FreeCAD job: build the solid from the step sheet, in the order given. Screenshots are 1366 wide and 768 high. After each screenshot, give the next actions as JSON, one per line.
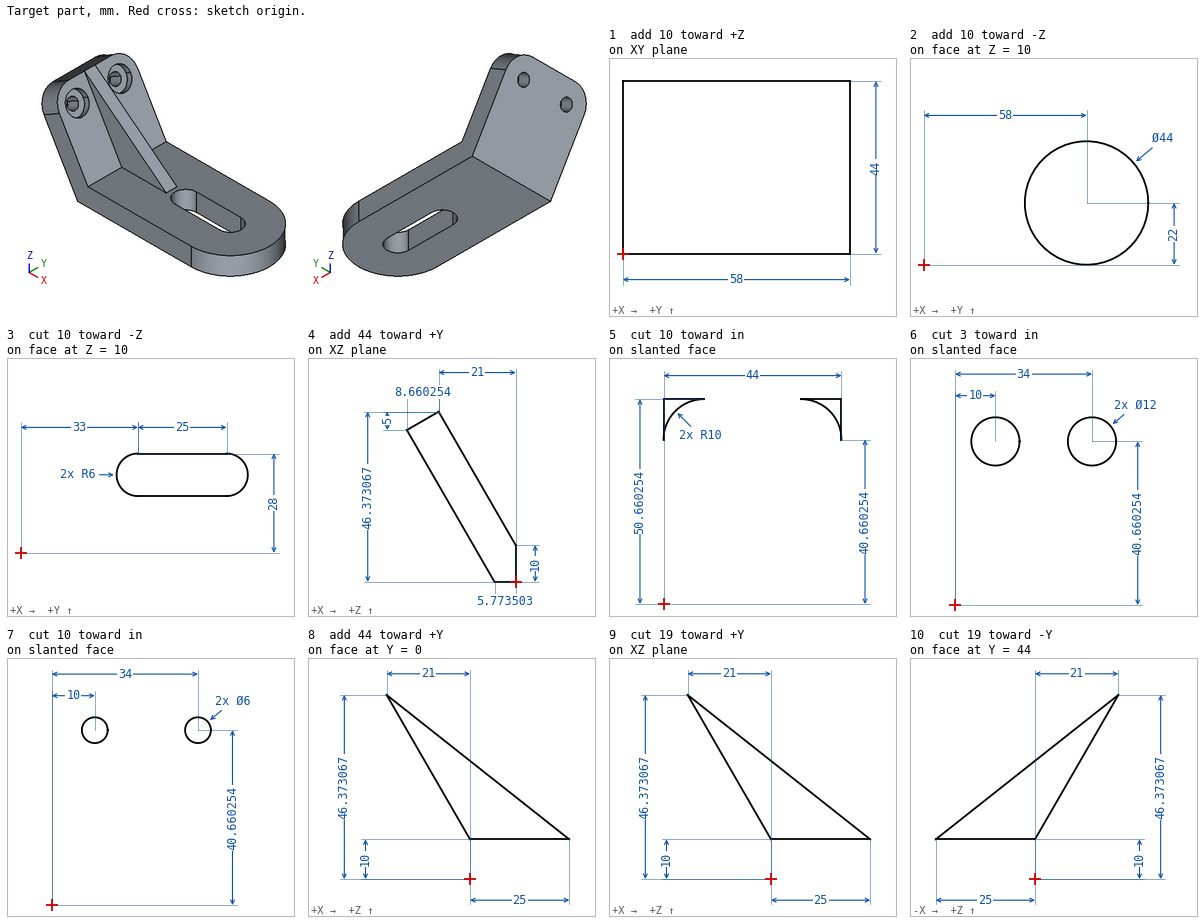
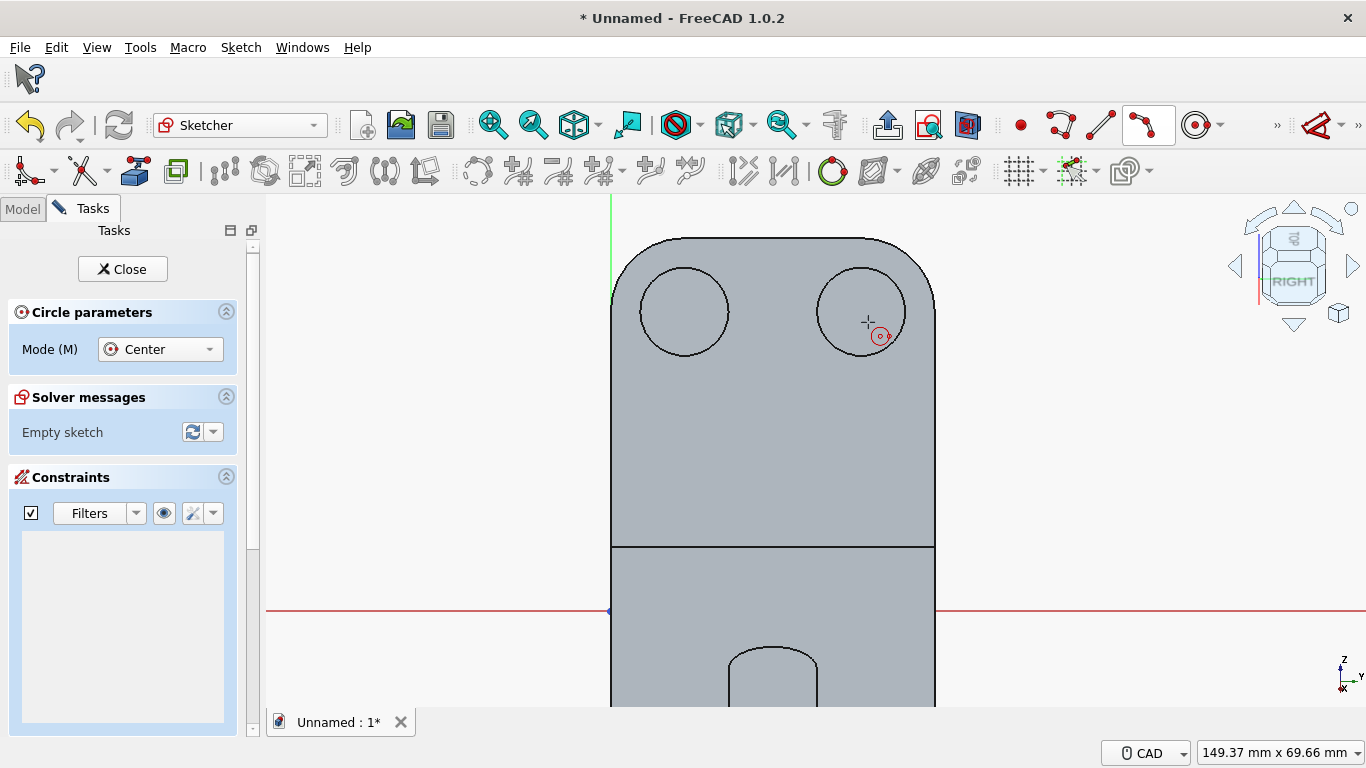
{"action": "left_click", "coordinate": [861, 312]}
{"action": "mouse_move", "coordinate": [877, 296]}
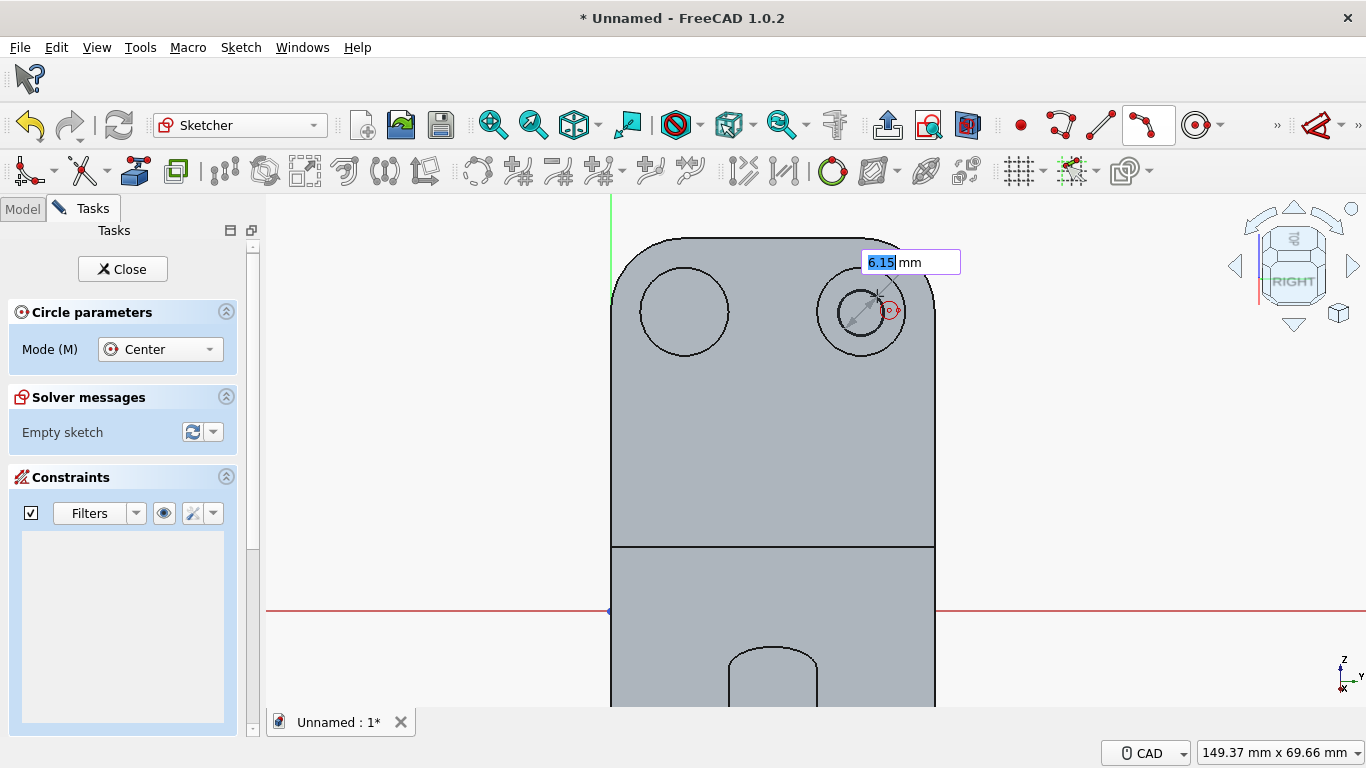
{"action": "type", "text": "6"}
{"action": "key", "text": "Return"}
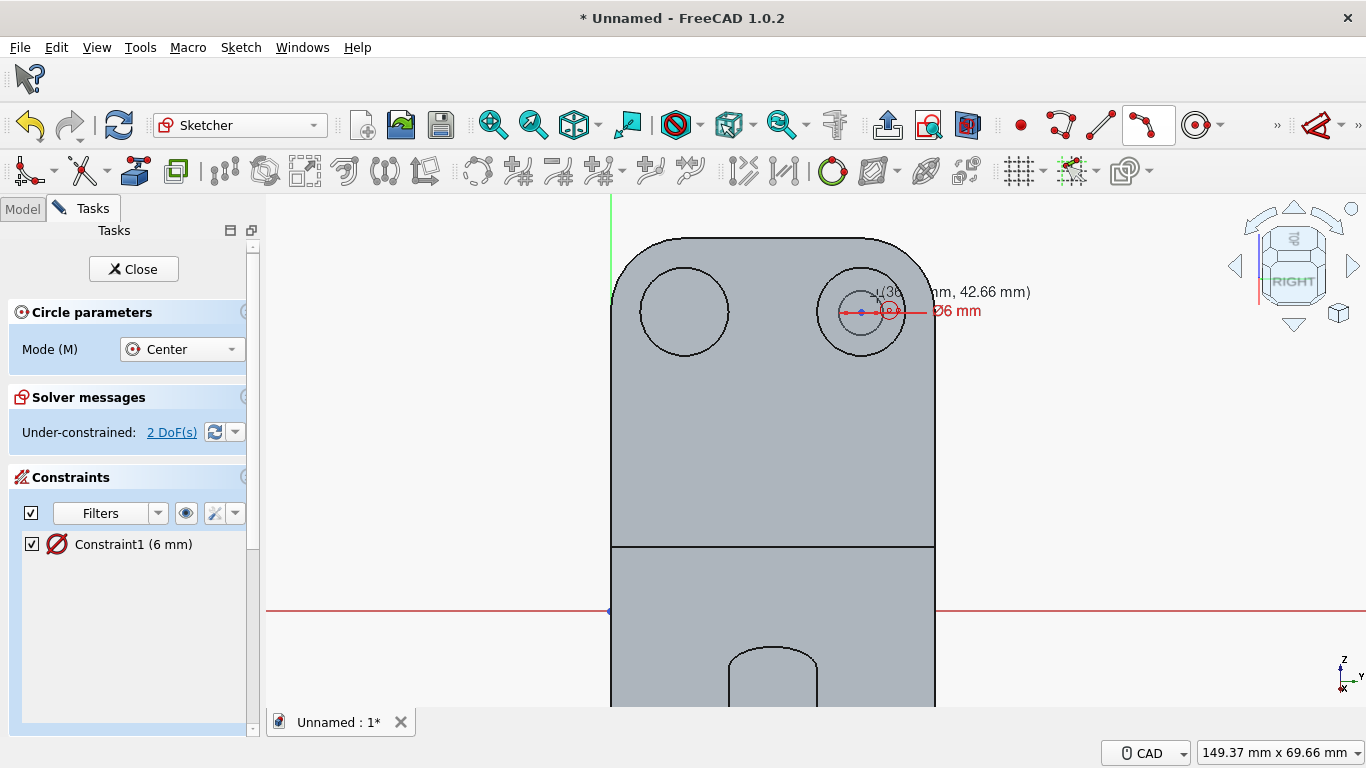
{"action": "left_click", "coordinate": [684, 312]}
{"action": "mouse_move", "coordinate": [700, 296]}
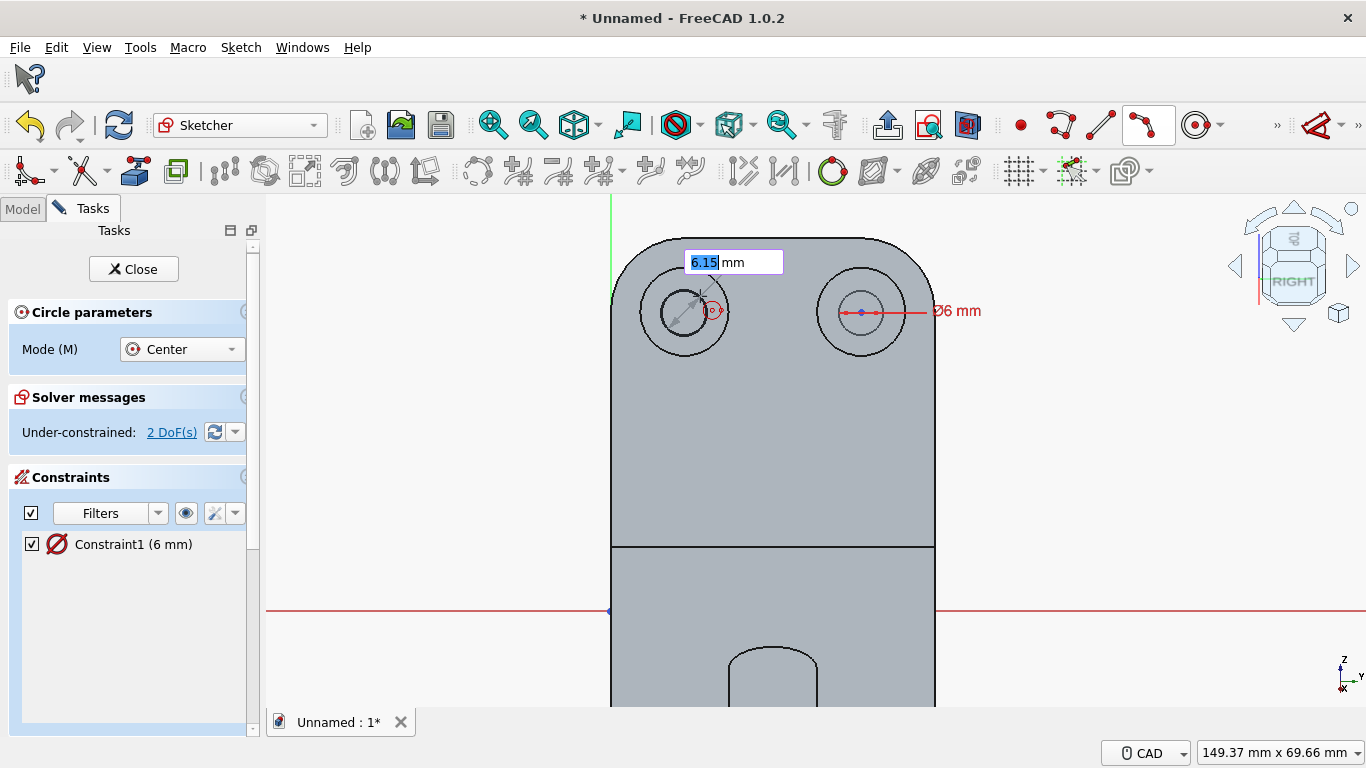
{"action": "type", "text": "6"}
{"action": "key", "text": "Return"}
{"action": "key", "text": "Escape"}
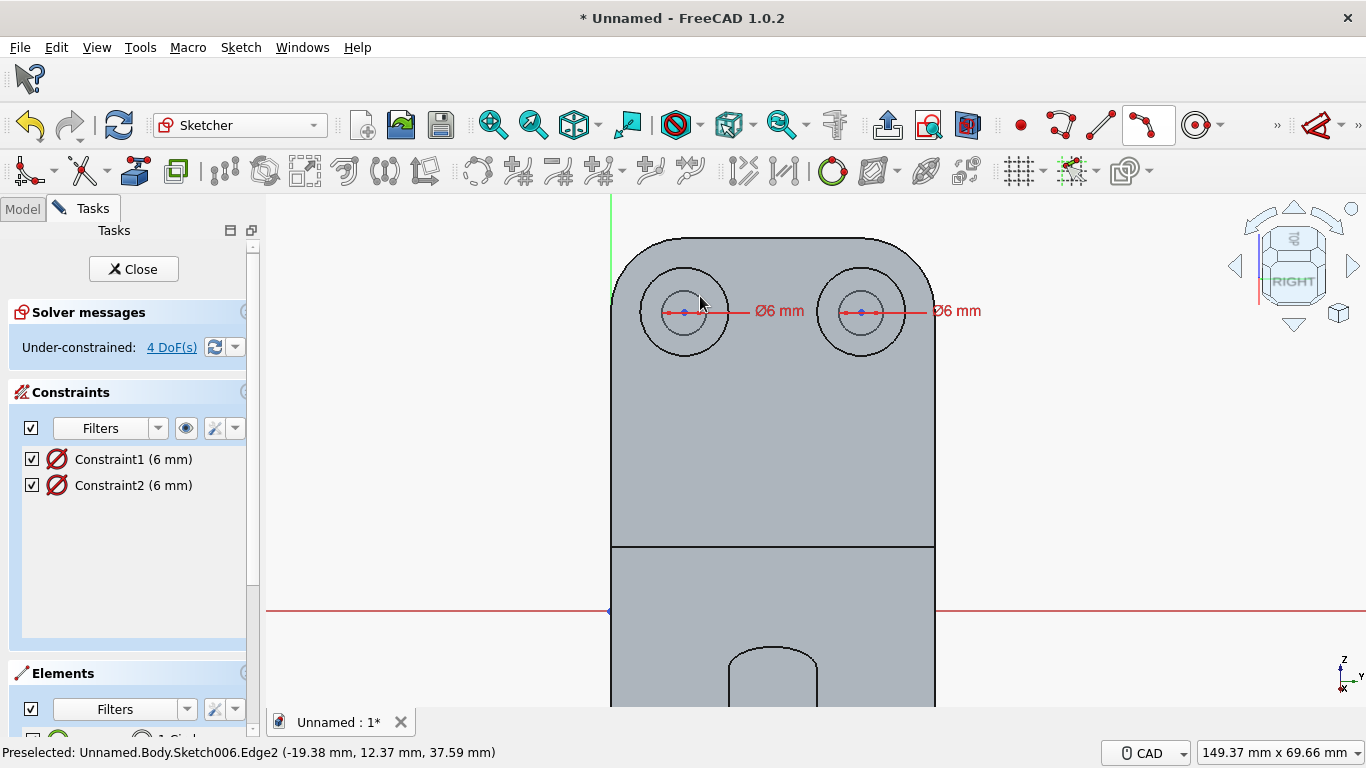
{"action": "left_click", "coordinate": [861, 313]}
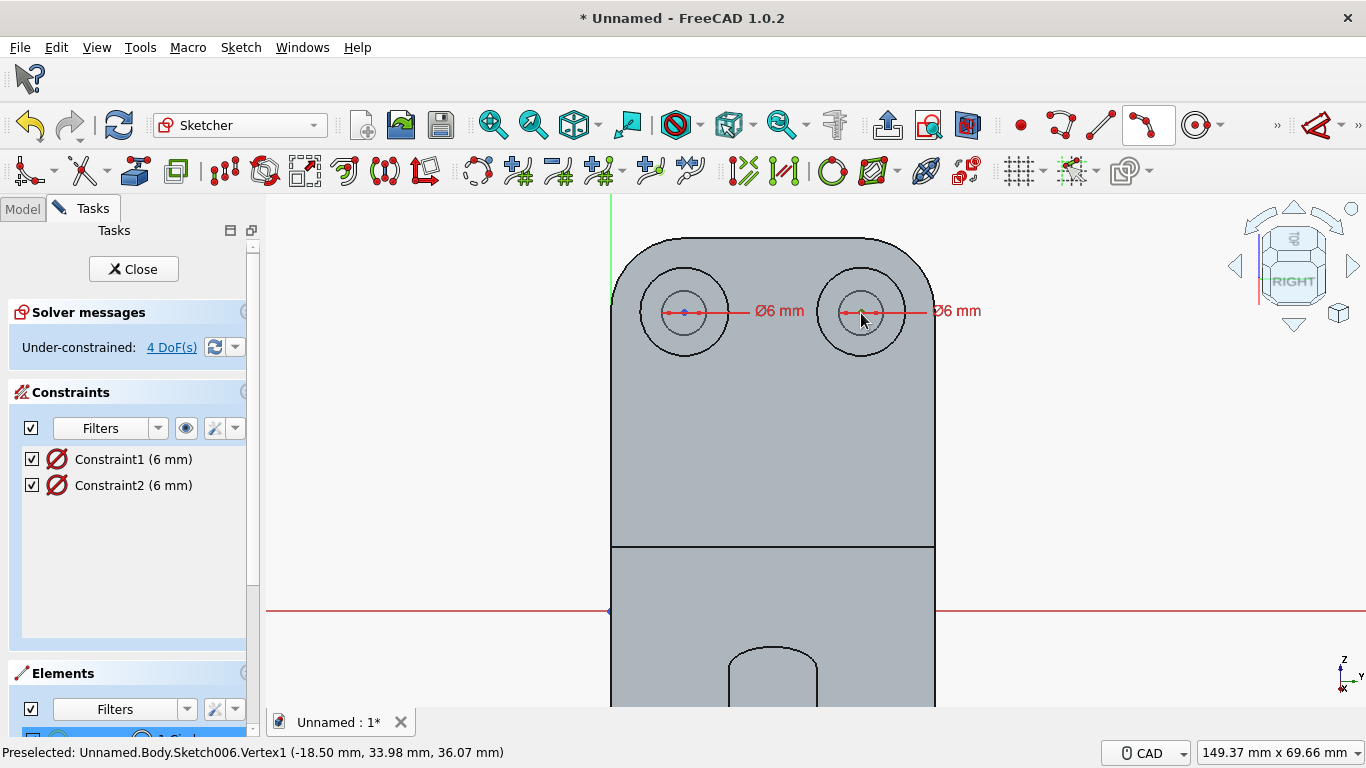
{"action": "left_click", "coordinate": [684, 313]}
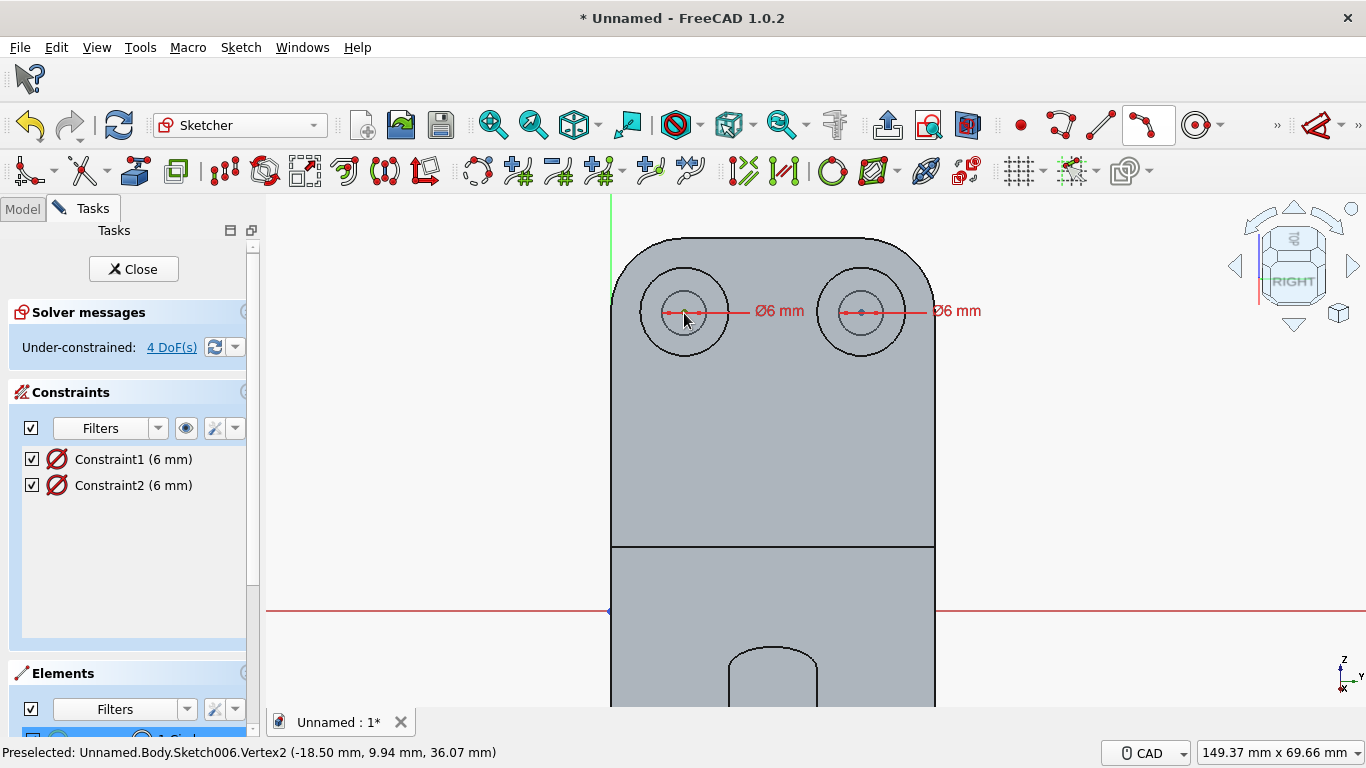
{"action": "key", "text": "h"}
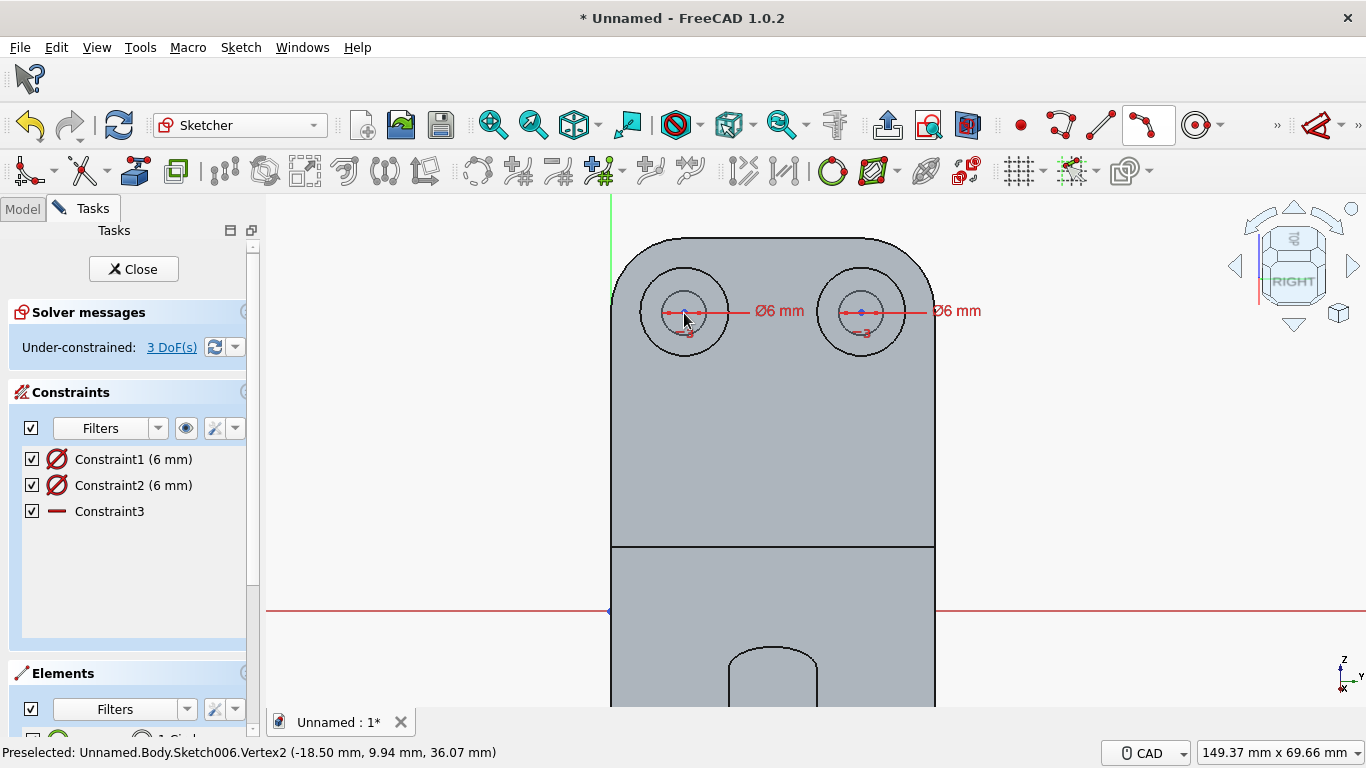
{"action": "left_click", "coordinate": [1316, 126]}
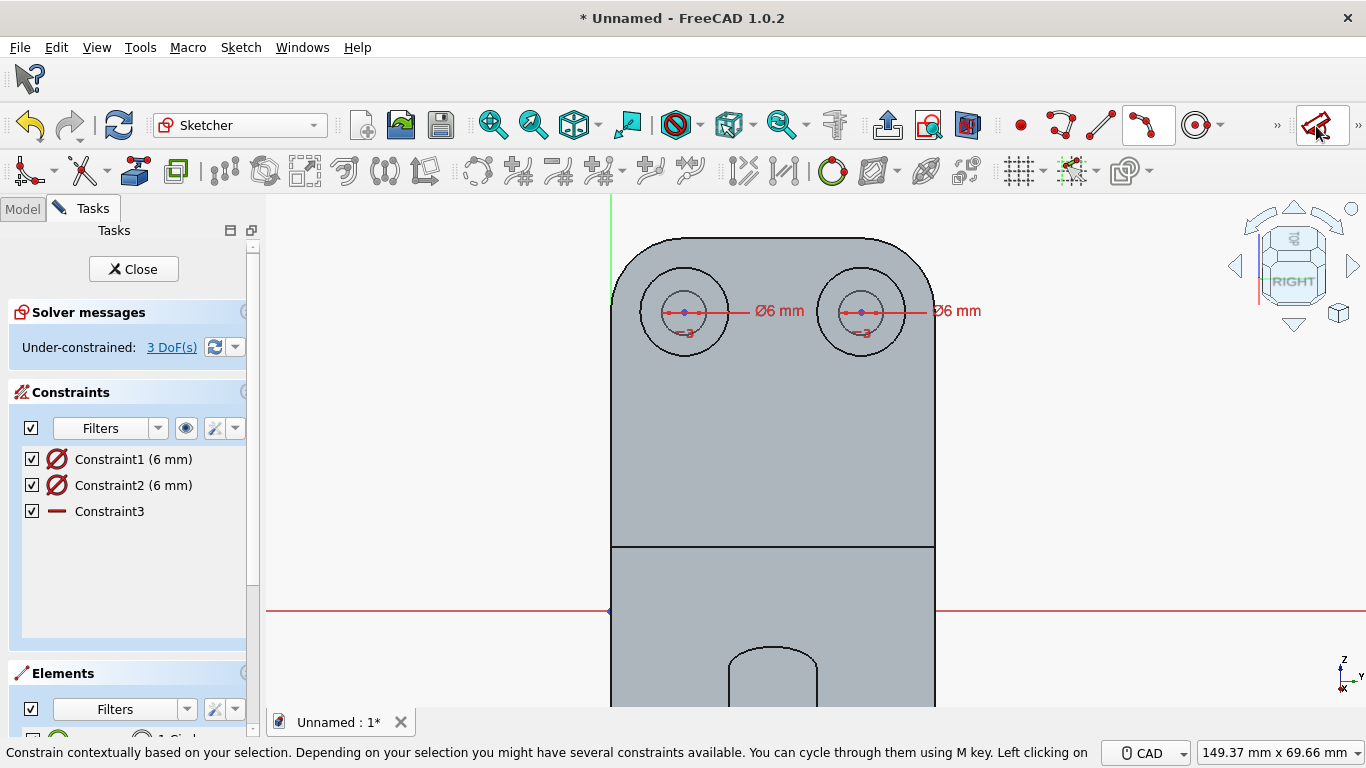
{"action": "left_click", "coordinate": [861, 313]}
{"action": "left_click", "coordinate": [736, 645]}